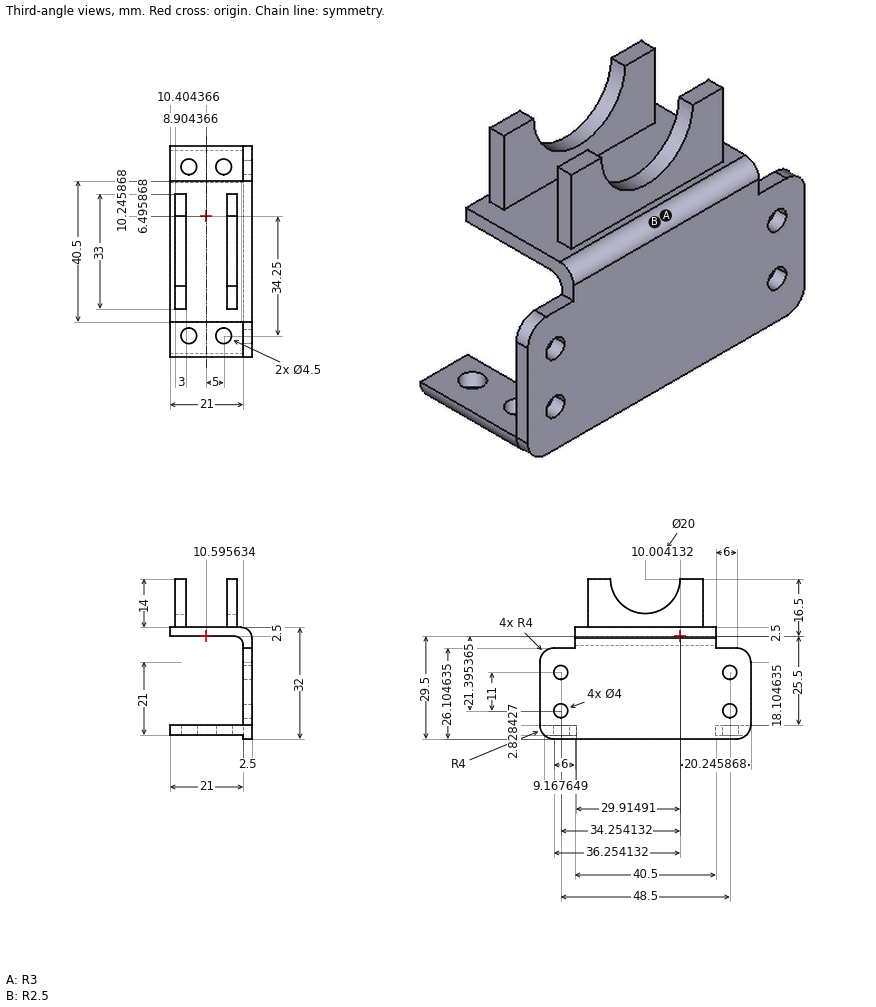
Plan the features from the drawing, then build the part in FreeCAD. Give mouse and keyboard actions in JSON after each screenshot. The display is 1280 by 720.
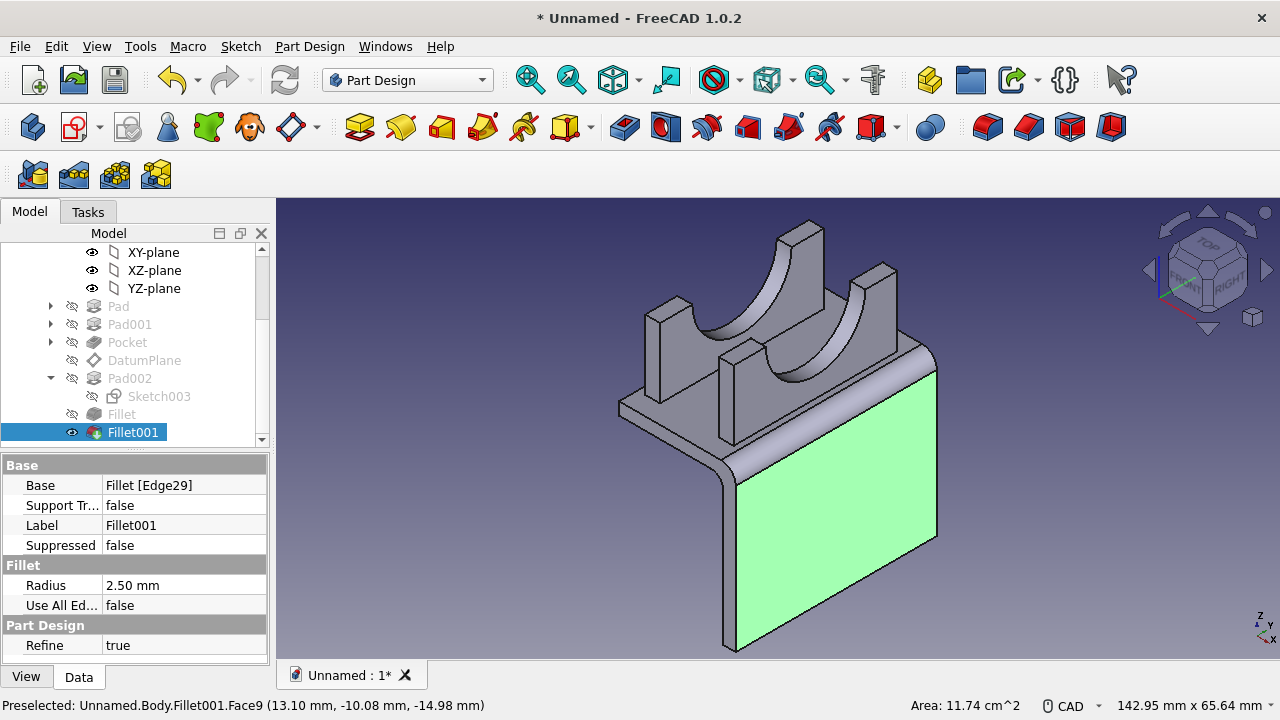
{"action": "left_click", "coordinate": [74, 128]}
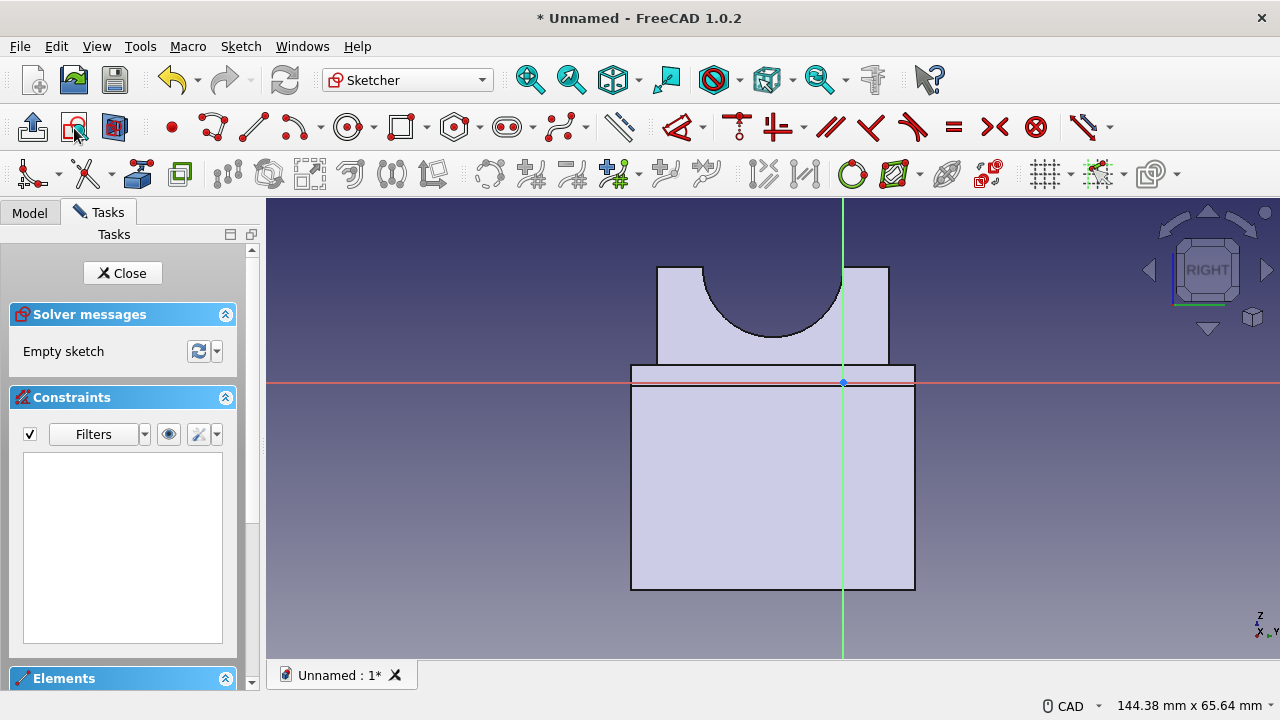
{"action": "scroll", "coordinate": [912, 604], "scroll_direction": "up", "scroll_amount": 2}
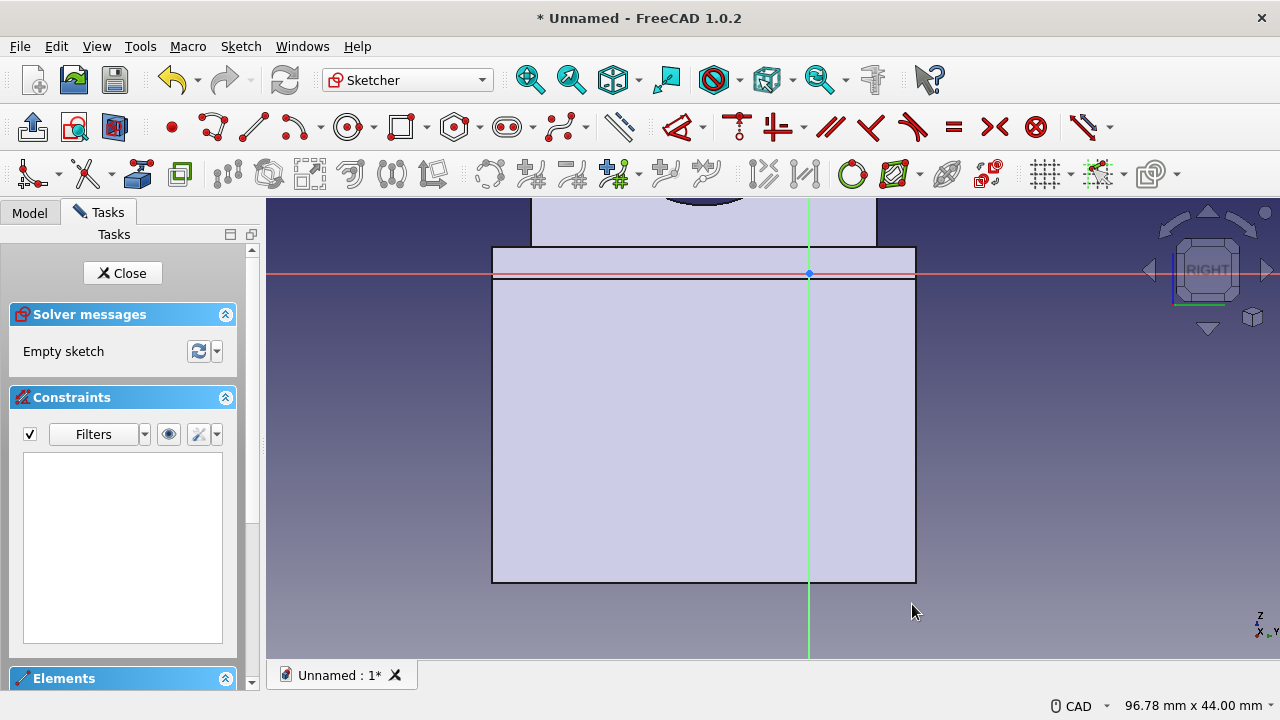
{"action": "left_click", "coordinate": [213, 128]}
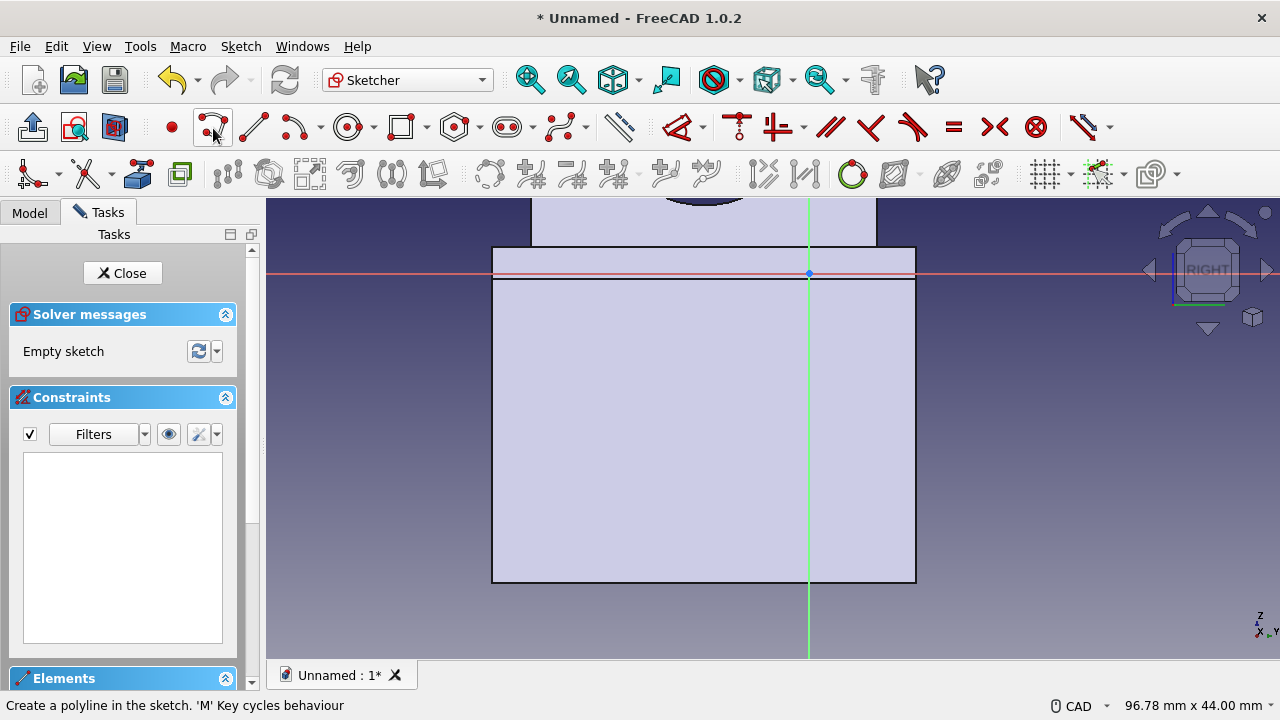
{"action": "left_click", "coordinate": [429, 583]}
{"action": "left_click", "coordinate": [492, 583]}
{"action": "left_click", "coordinate": [492, 309]}
{"action": "left_click", "coordinate": [429, 309]}
{"action": "right_click", "coordinate": [429, 309]}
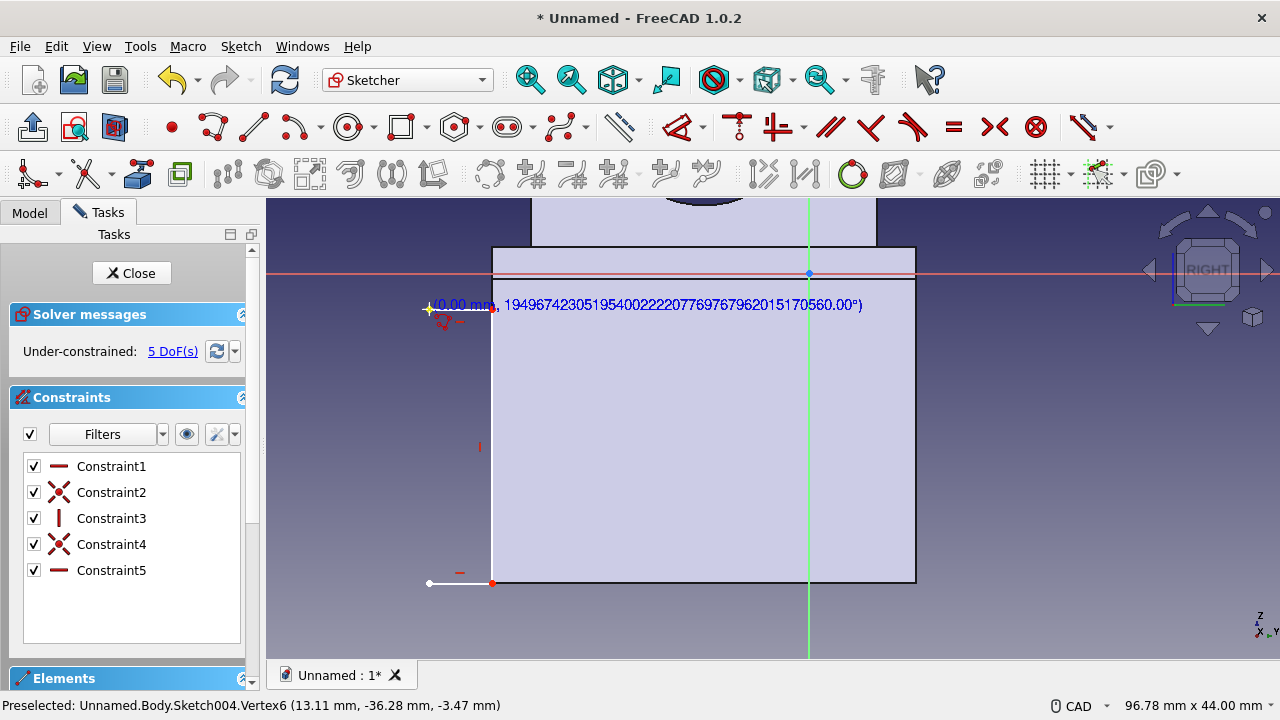
{"action": "left_click", "coordinate": [254, 128]}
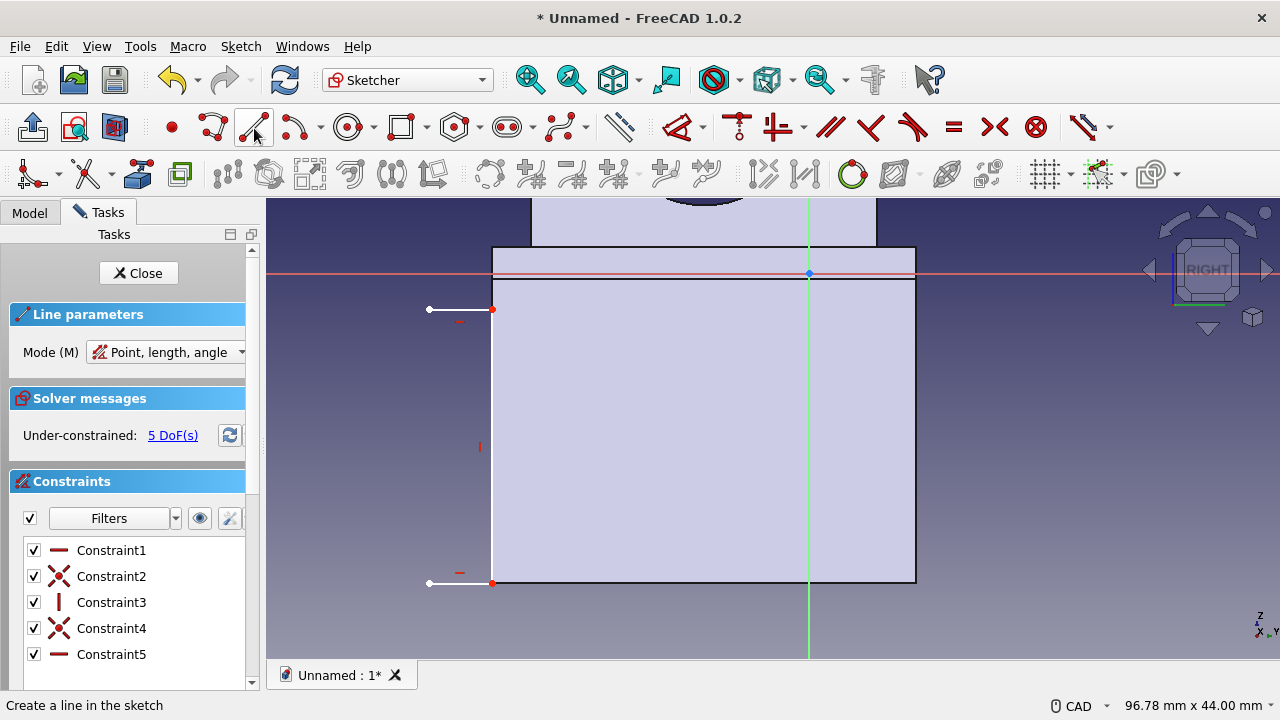
{"action": "left_click", "coordinate": [387, 351]}
{"action": "left_click", "coordinate": [387, 541]}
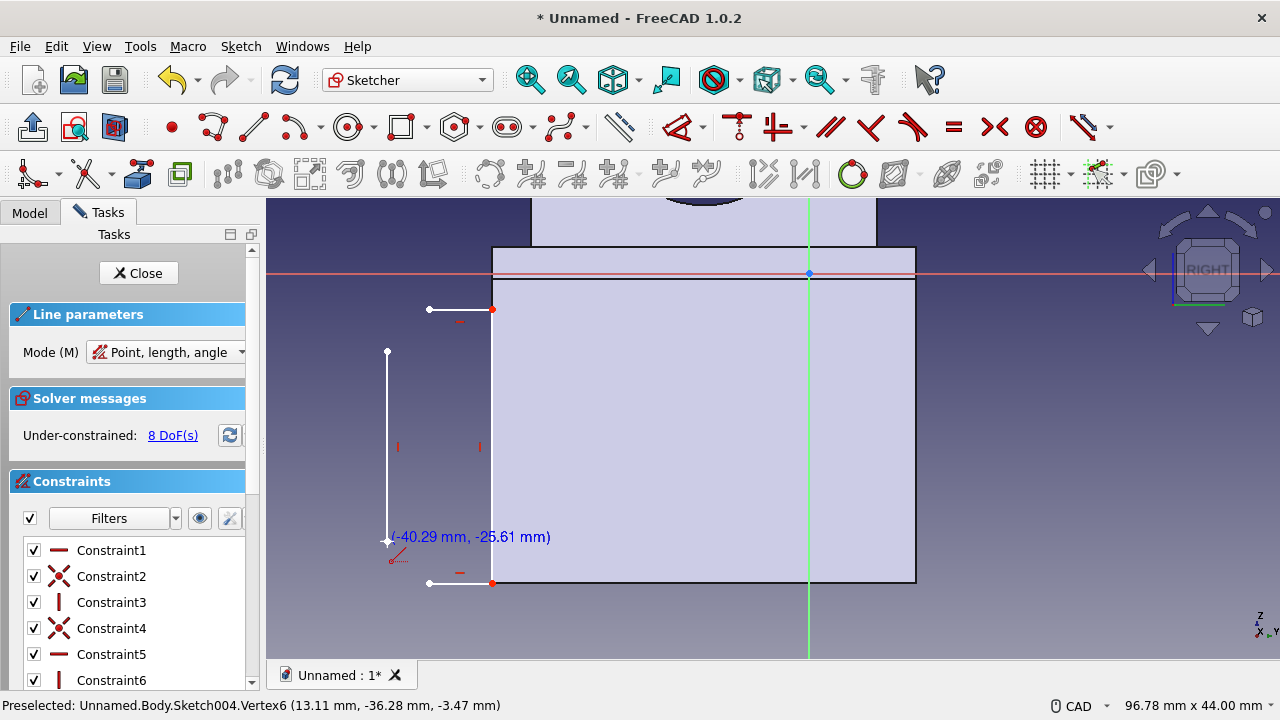
{"action": "key", "text": "g 3 a"}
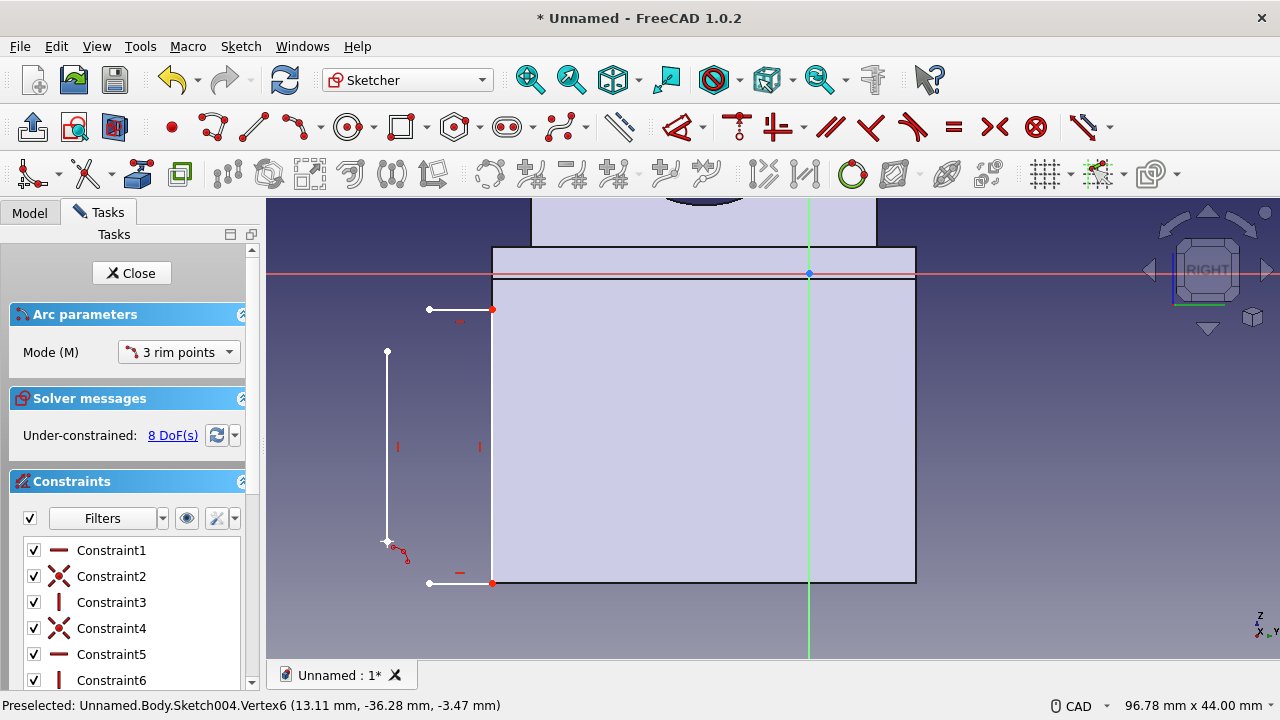
{"action": "left_click", "coordinate": [429, 310]}
{"action": "left_click", "coordinate": [387, 352]}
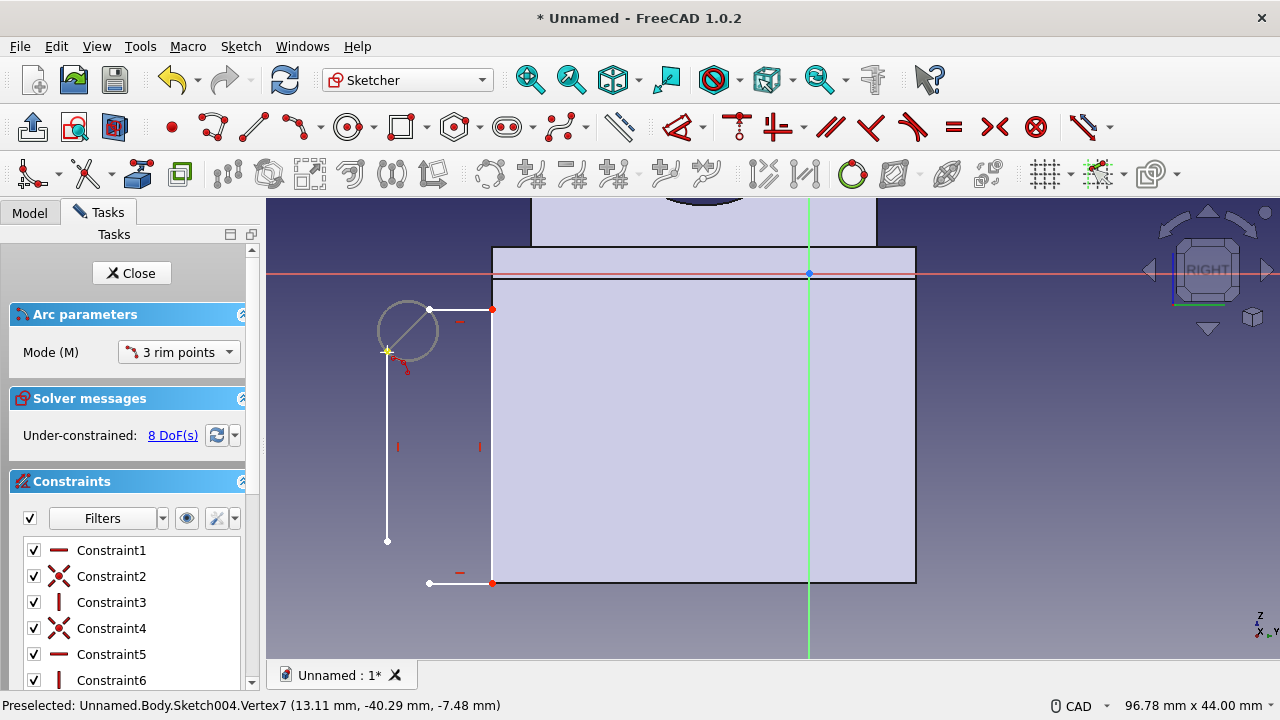
{"action": "scroll", "coordinate": [400, 321], "scroll_direction": "up", "scroll_amount": 2}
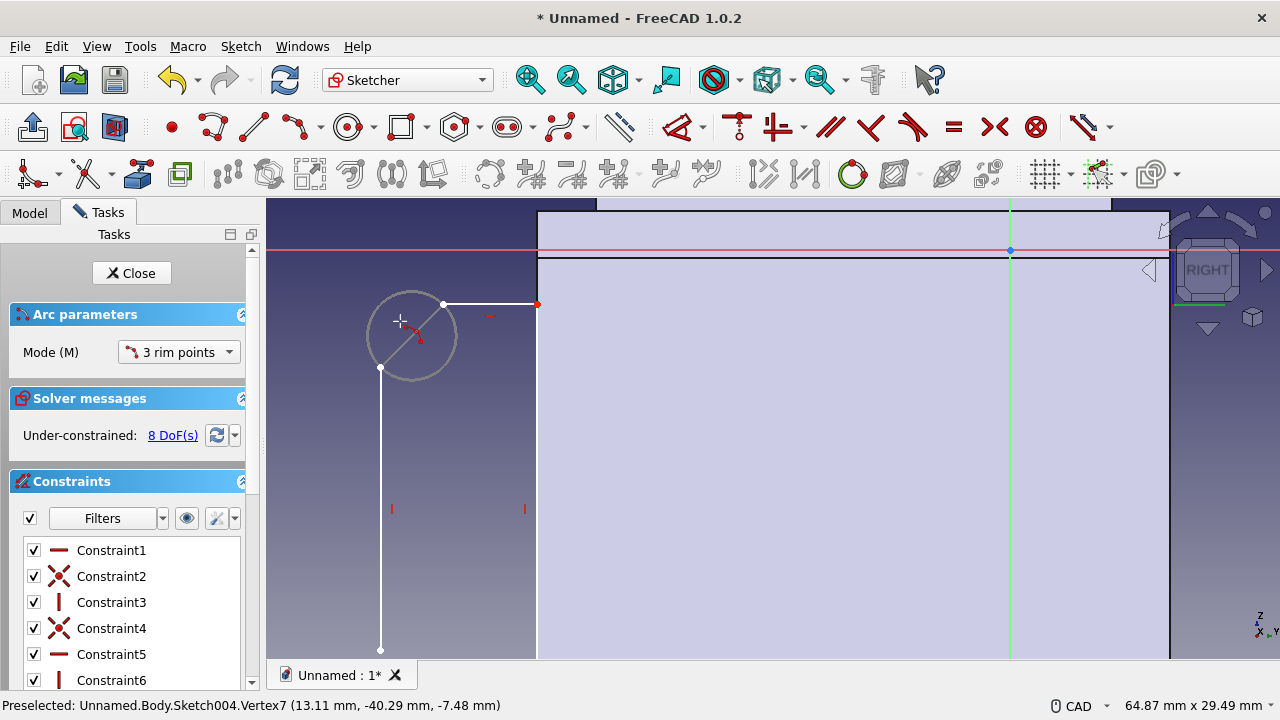
{"action": "left_click", "coordinate": [399, 322]}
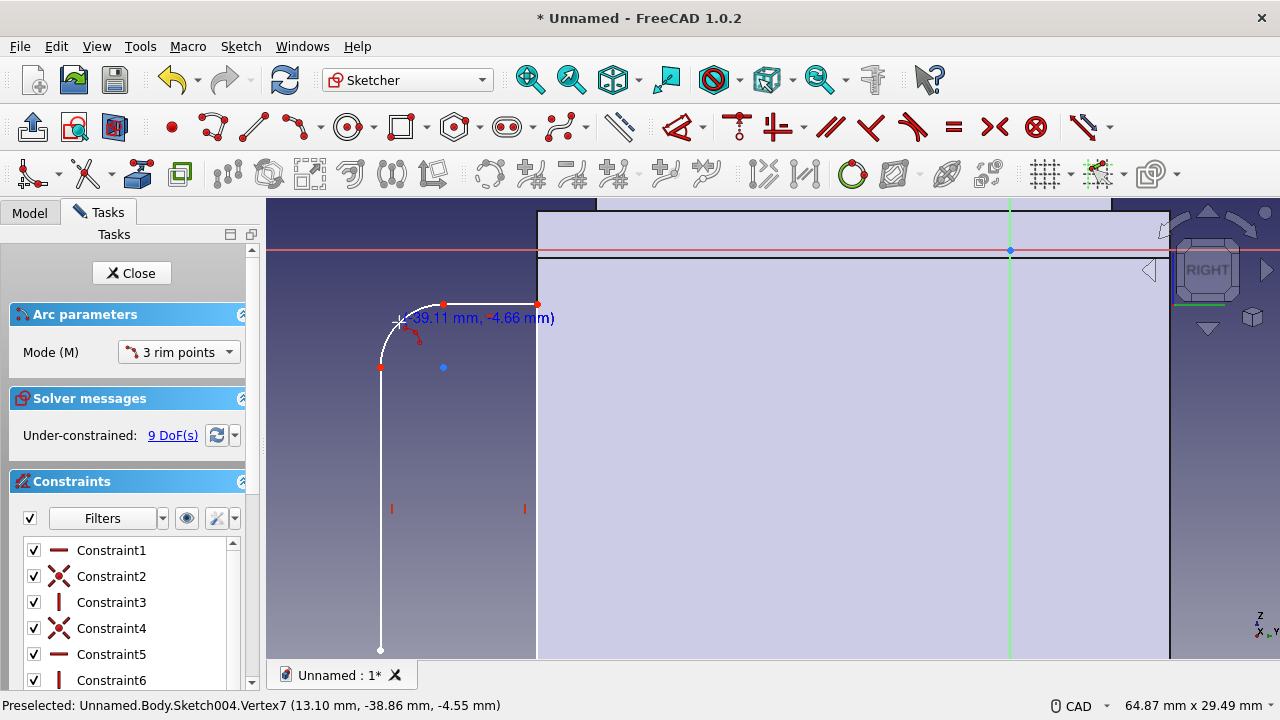
{"action": "scroll", "coordinate": [401, 322], "scroll_direction": "down", "scroll_amount": 2}